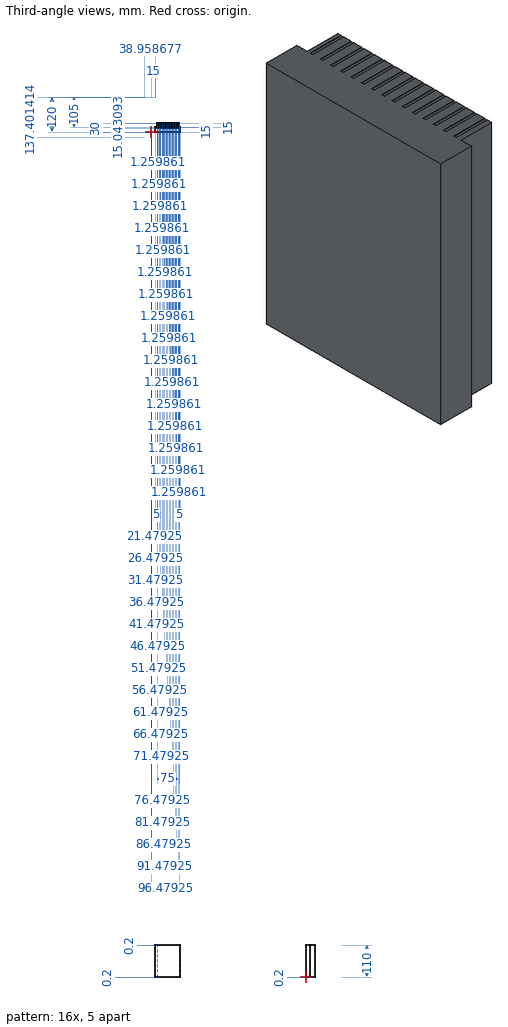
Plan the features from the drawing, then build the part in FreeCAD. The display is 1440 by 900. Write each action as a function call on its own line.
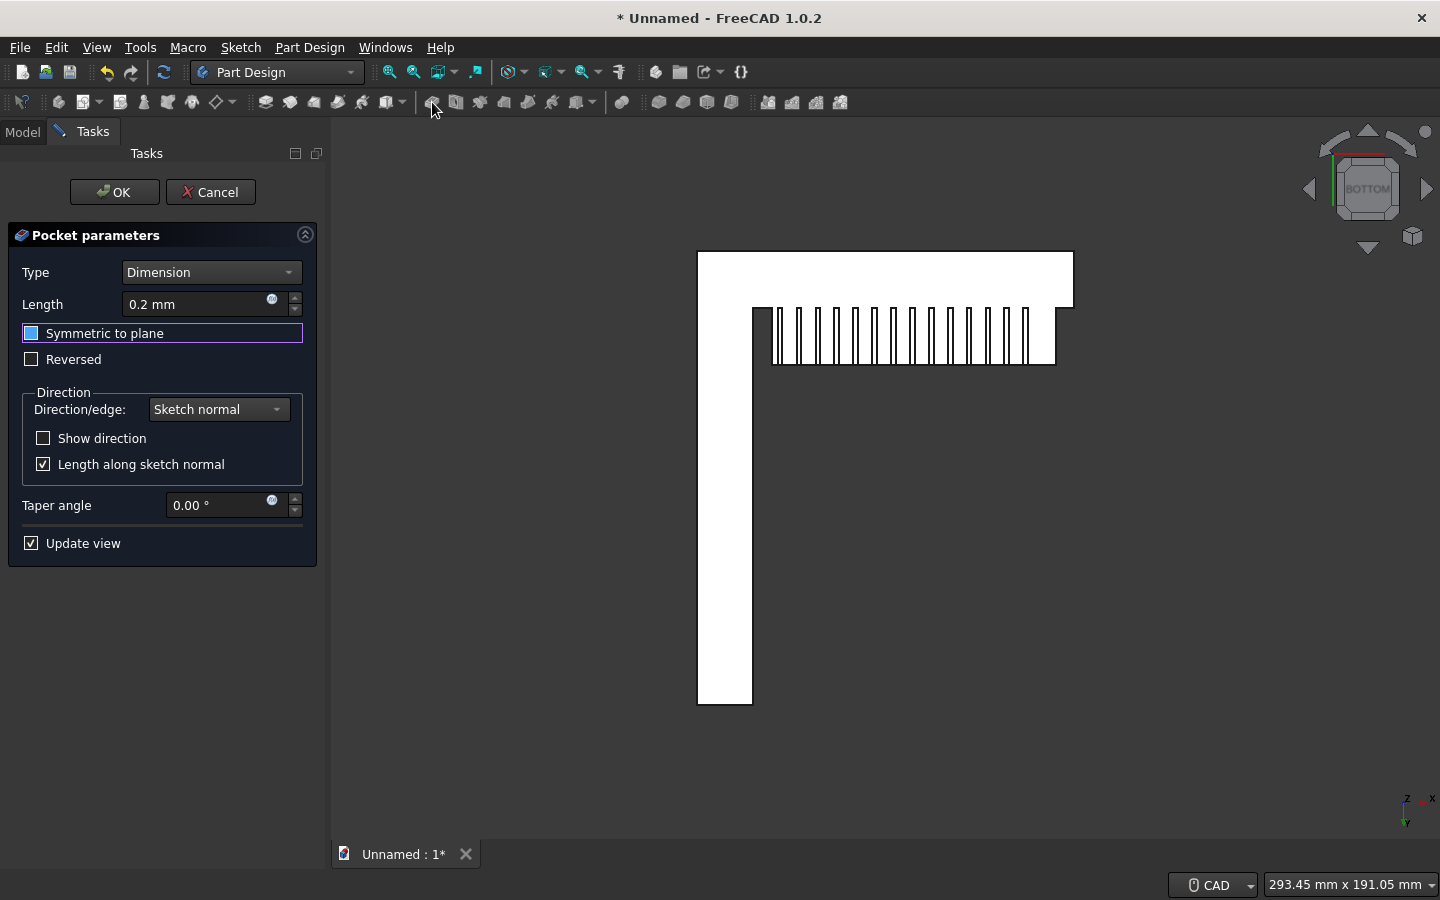
click(30, 359)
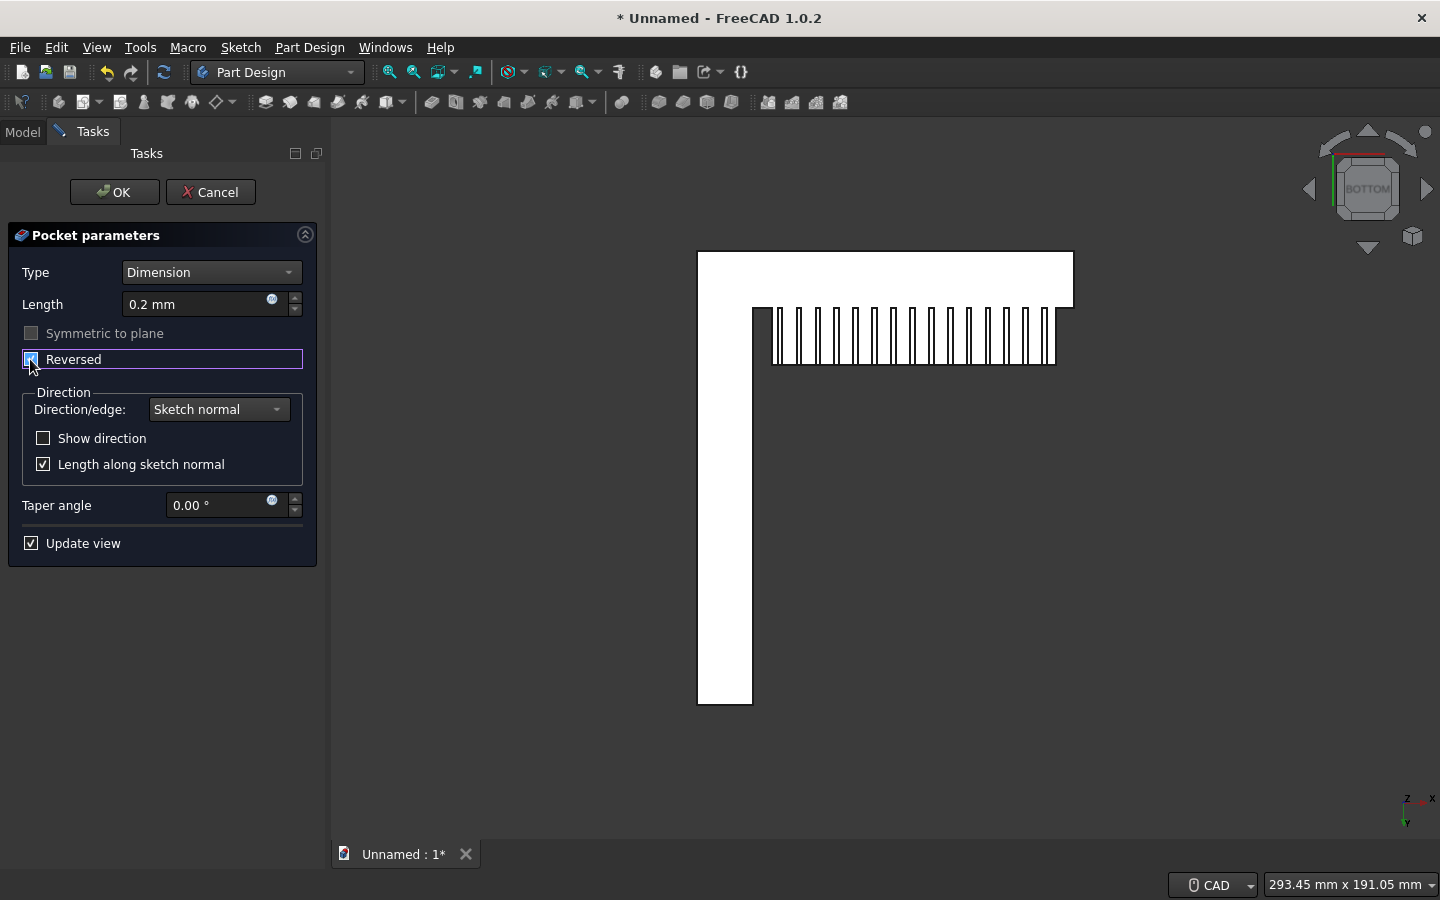
click(115, 192)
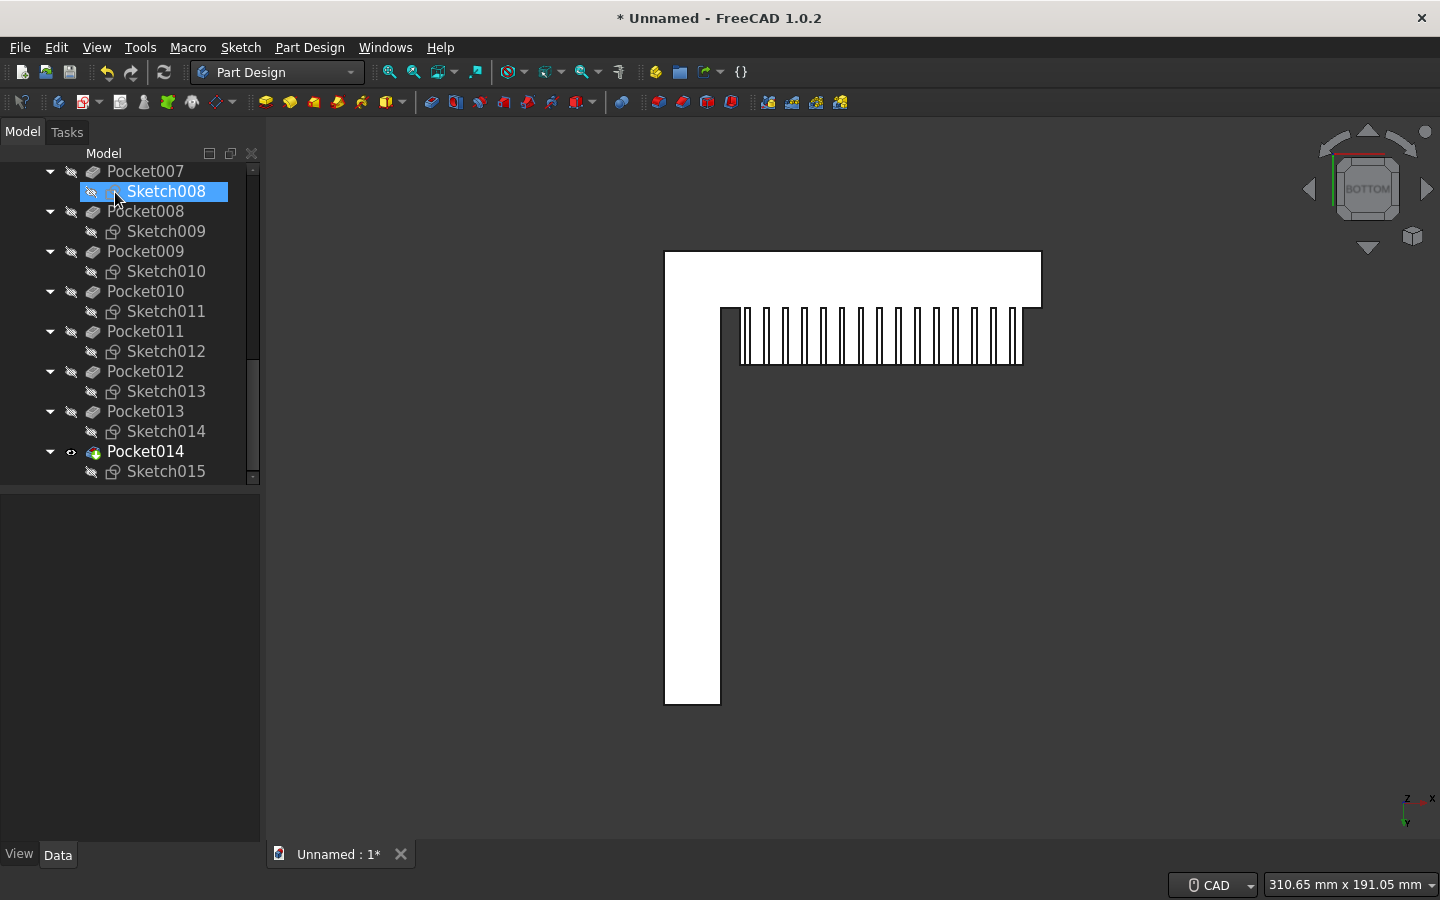
click(691, 671)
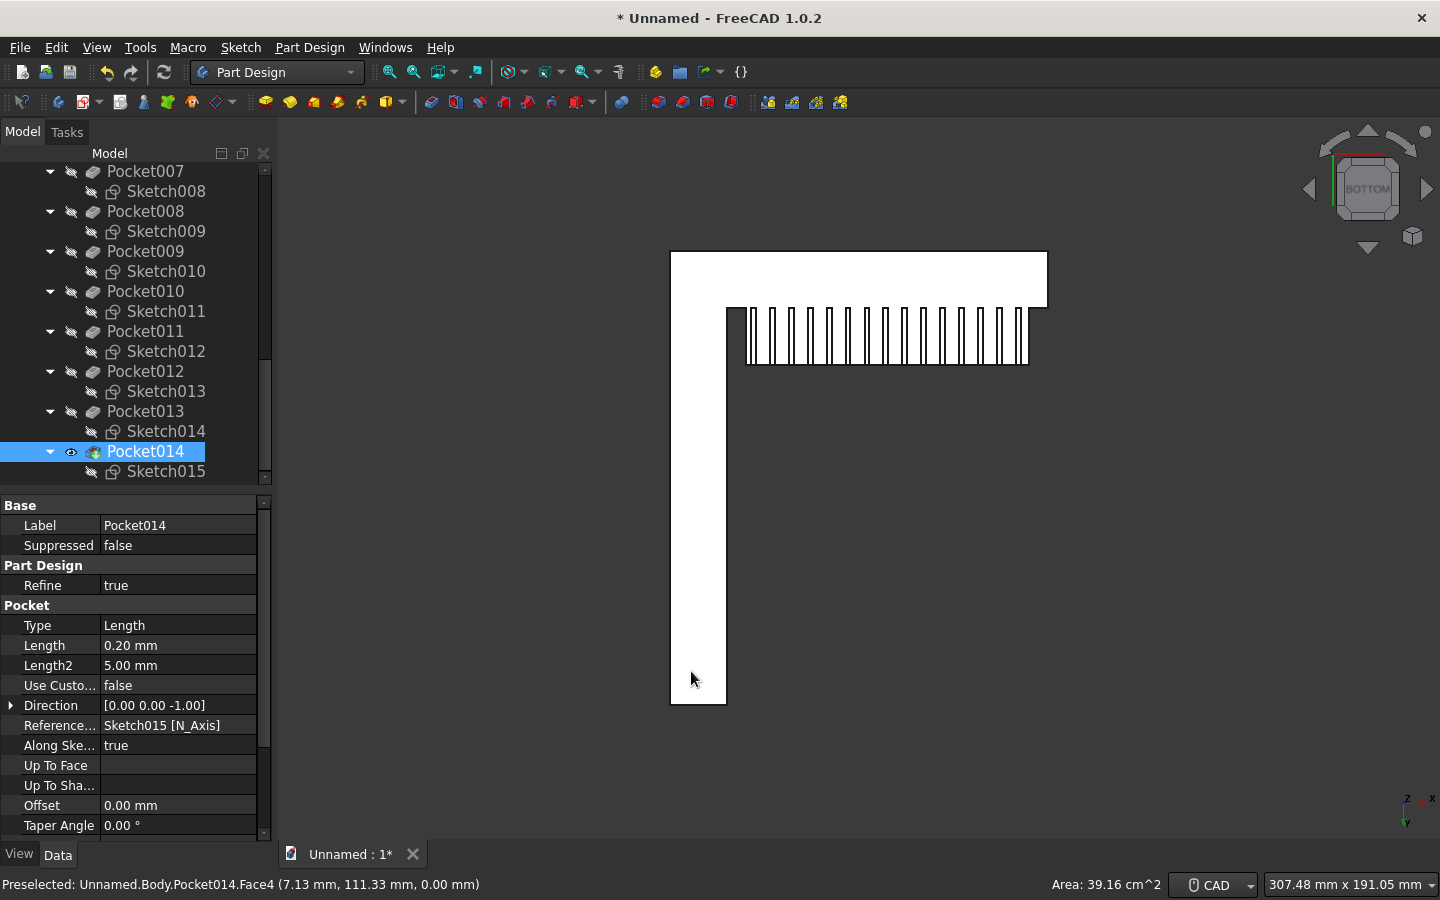
click(84, 102)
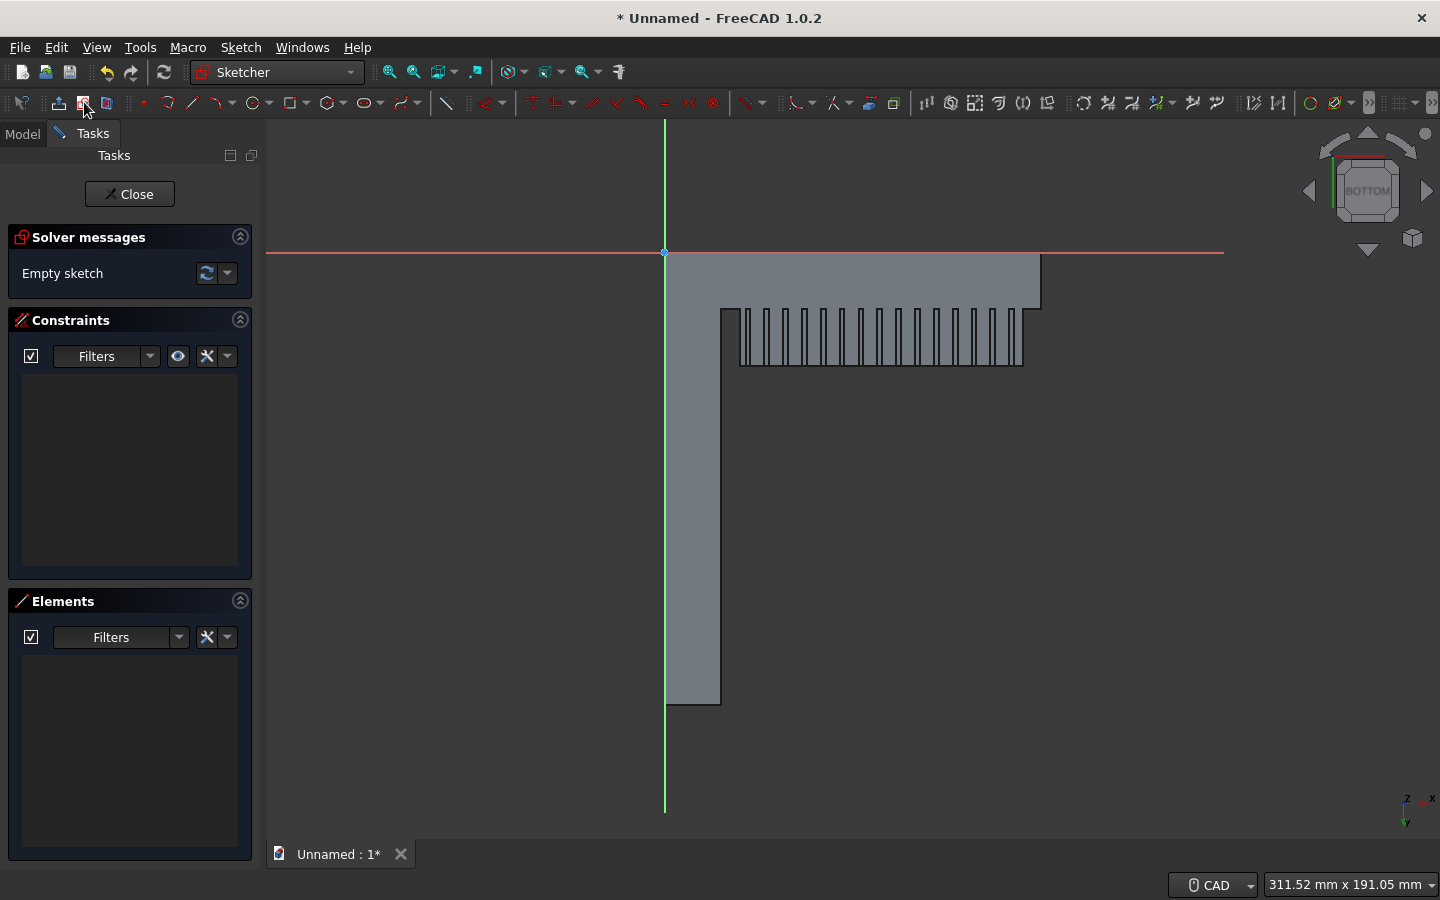
scroll(1061, 320, up, 11)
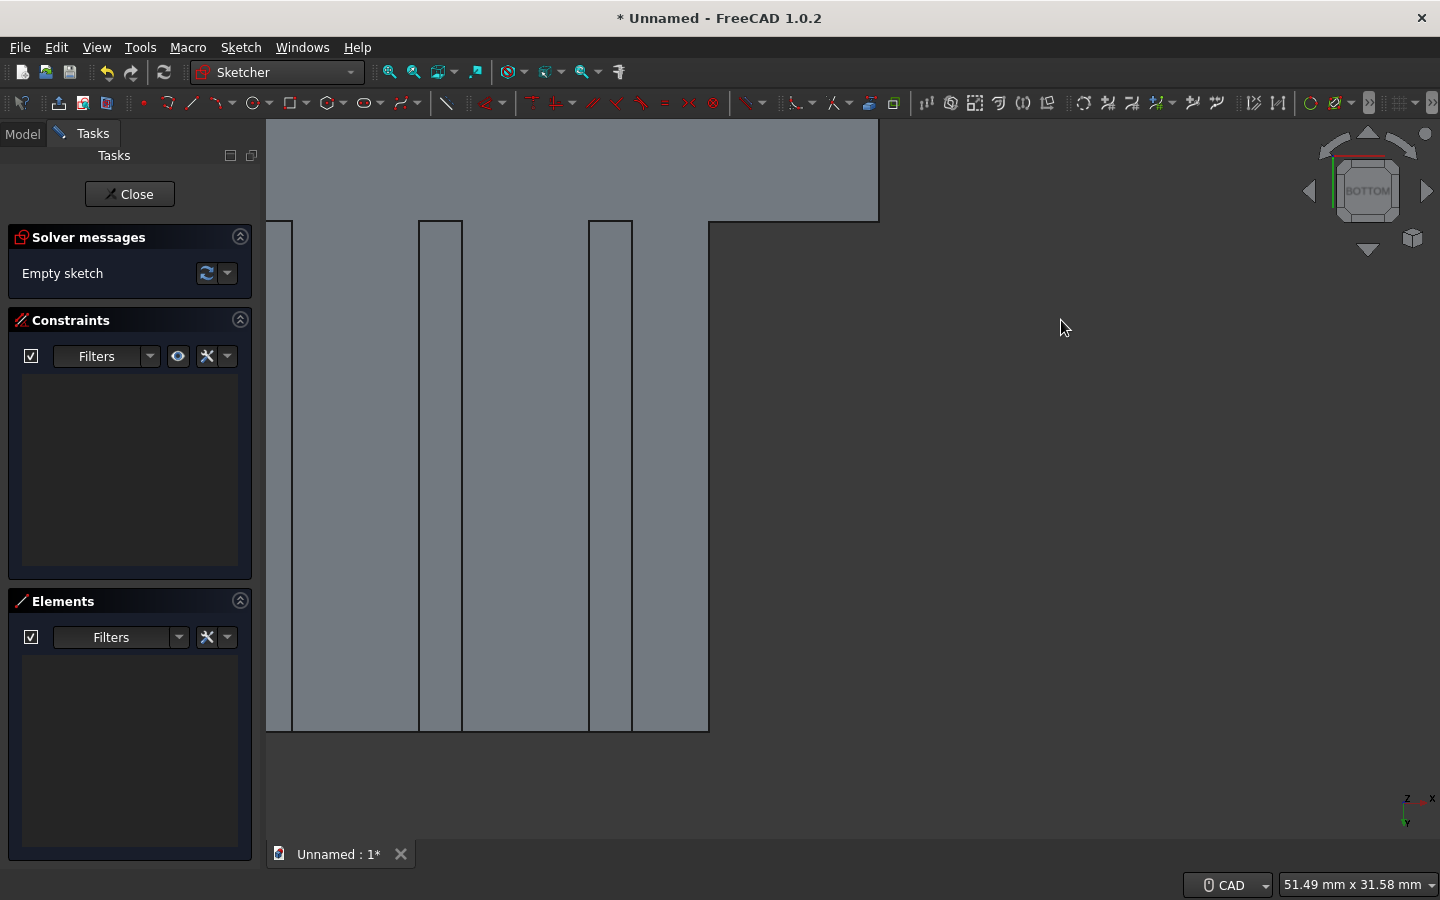
click(290, 104)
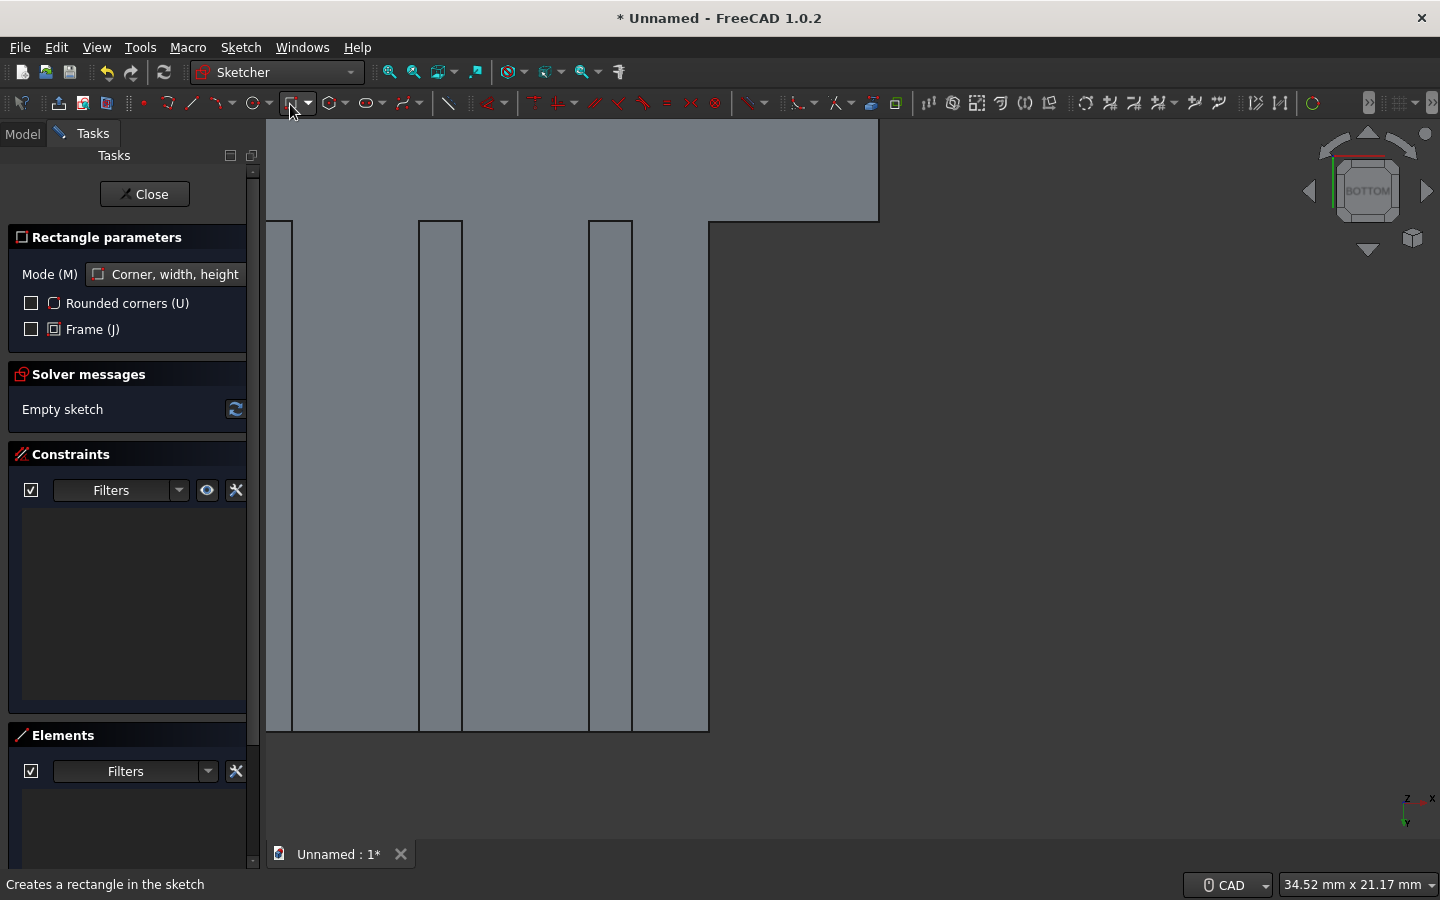
click(759, 221)
click(802, 732)
key(Escape)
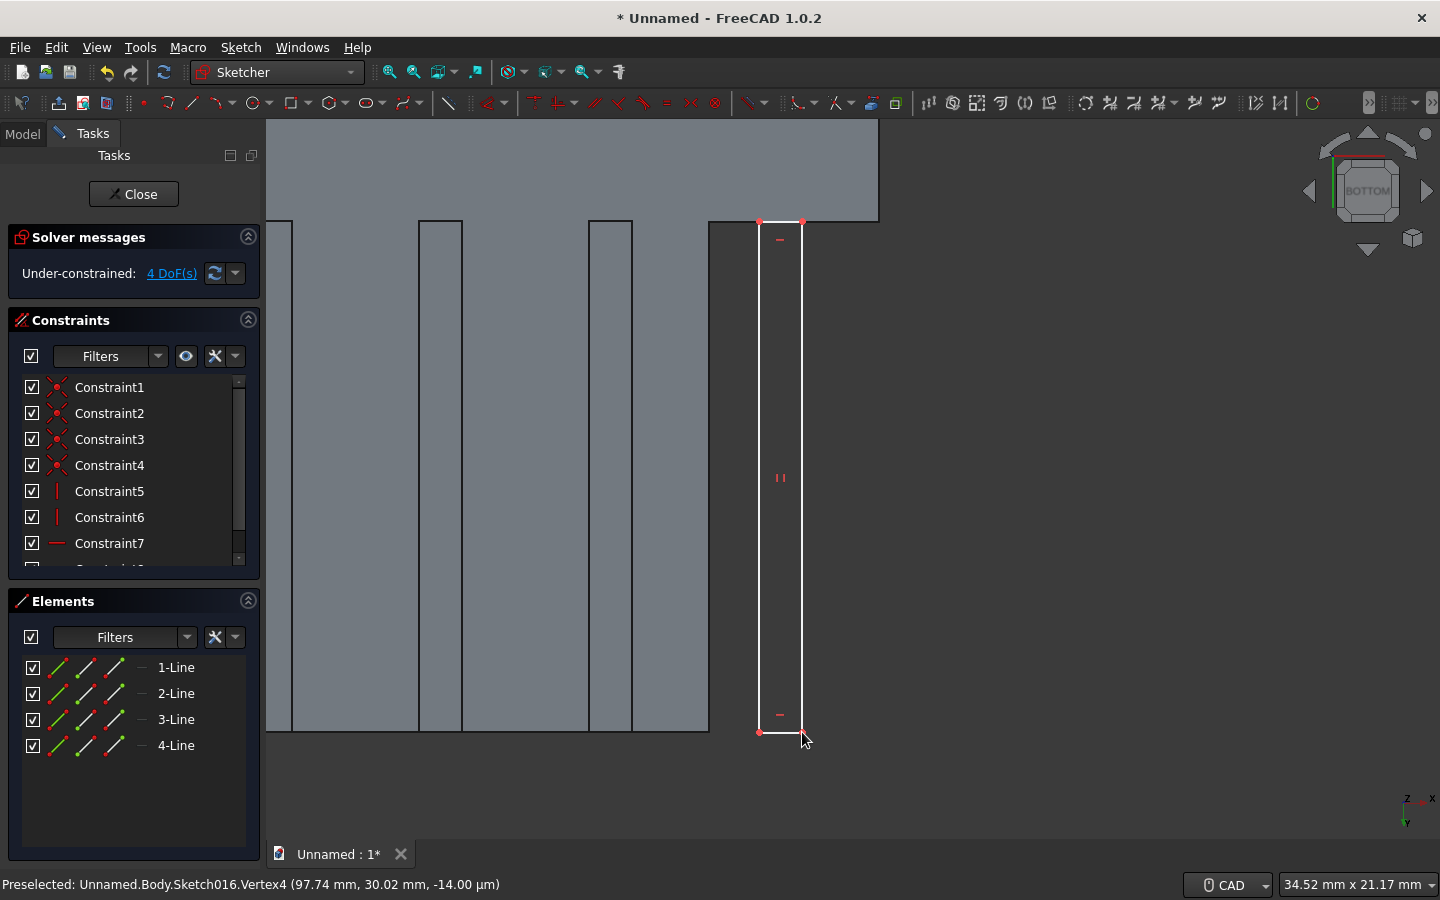
click(488, 104)